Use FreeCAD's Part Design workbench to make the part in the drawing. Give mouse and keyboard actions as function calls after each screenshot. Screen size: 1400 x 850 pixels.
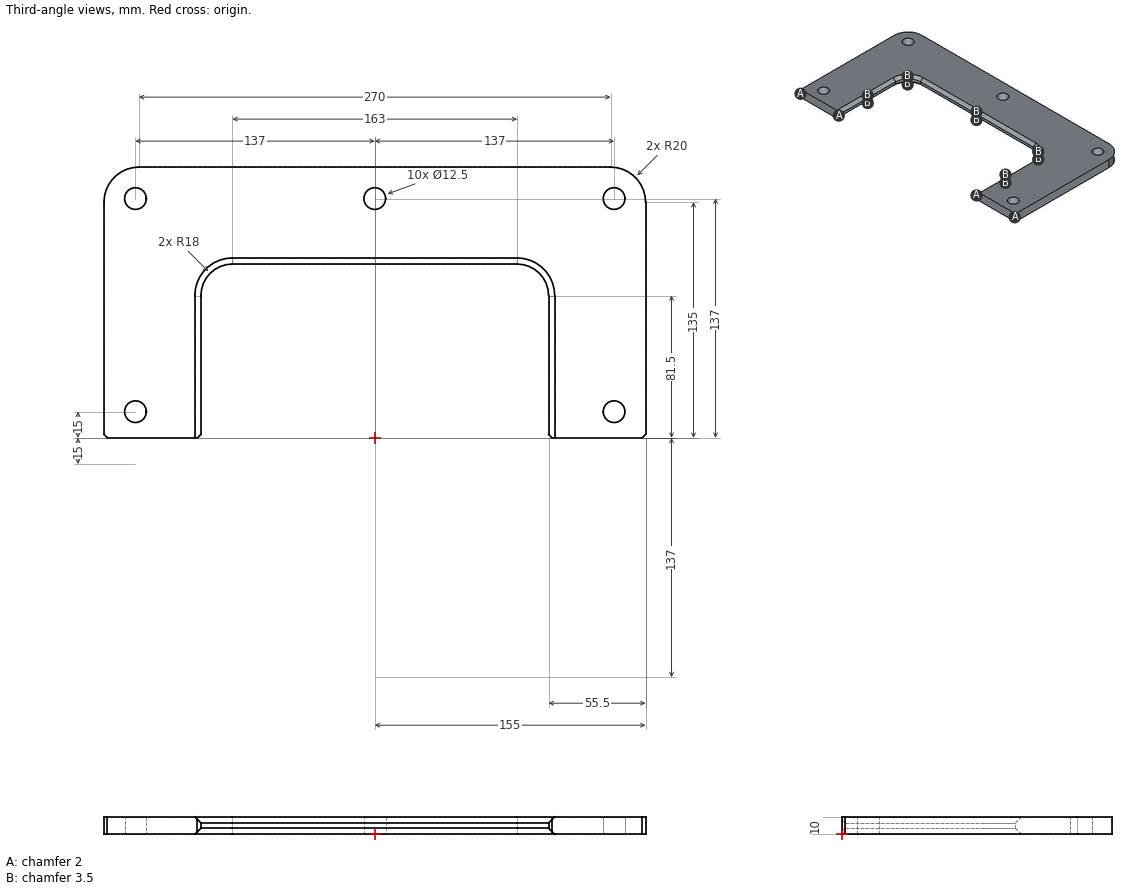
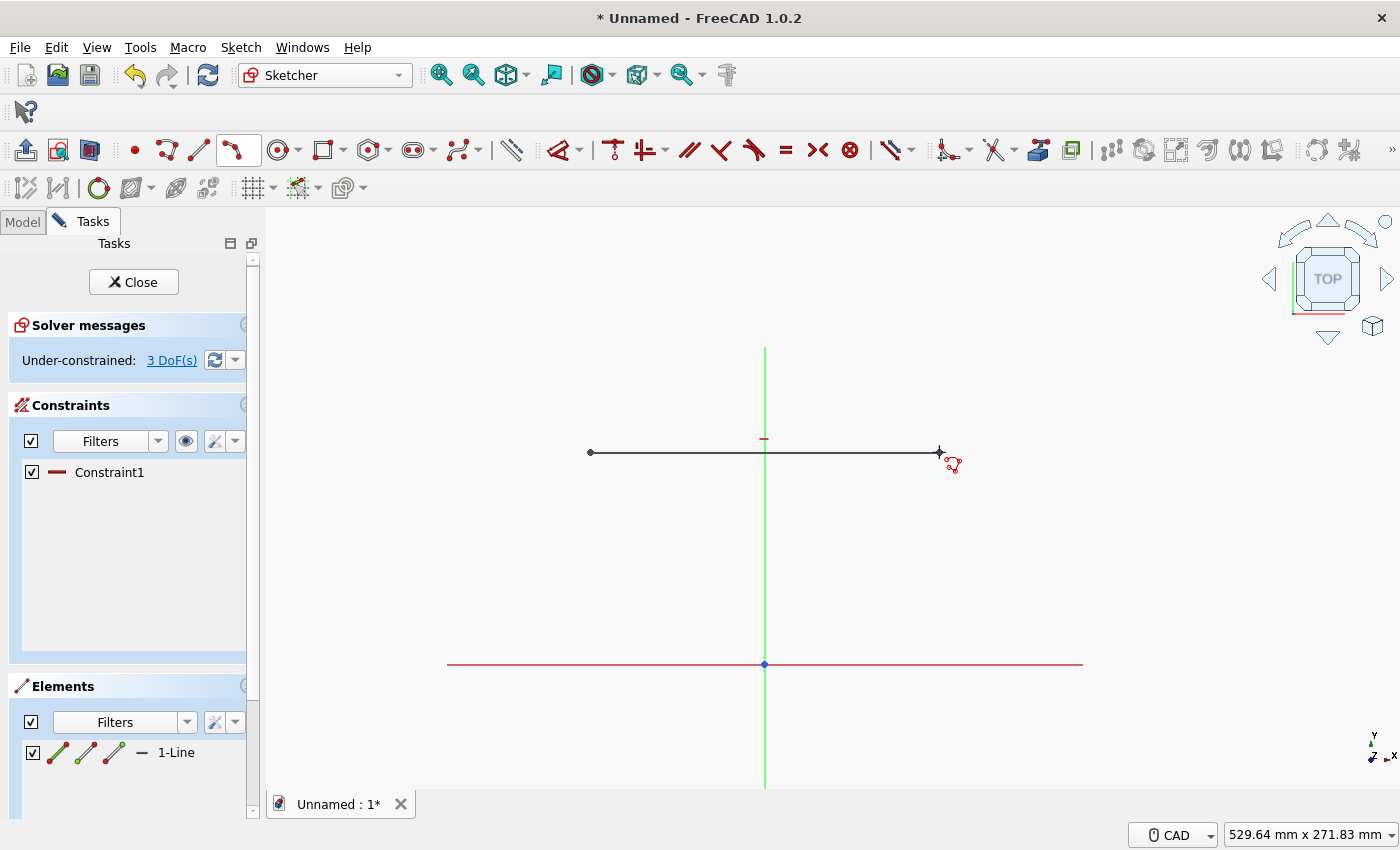
click(978, 490)
click(978, 665)
click(1097, 656)
click(1097, 376)
right_click(1097, 376)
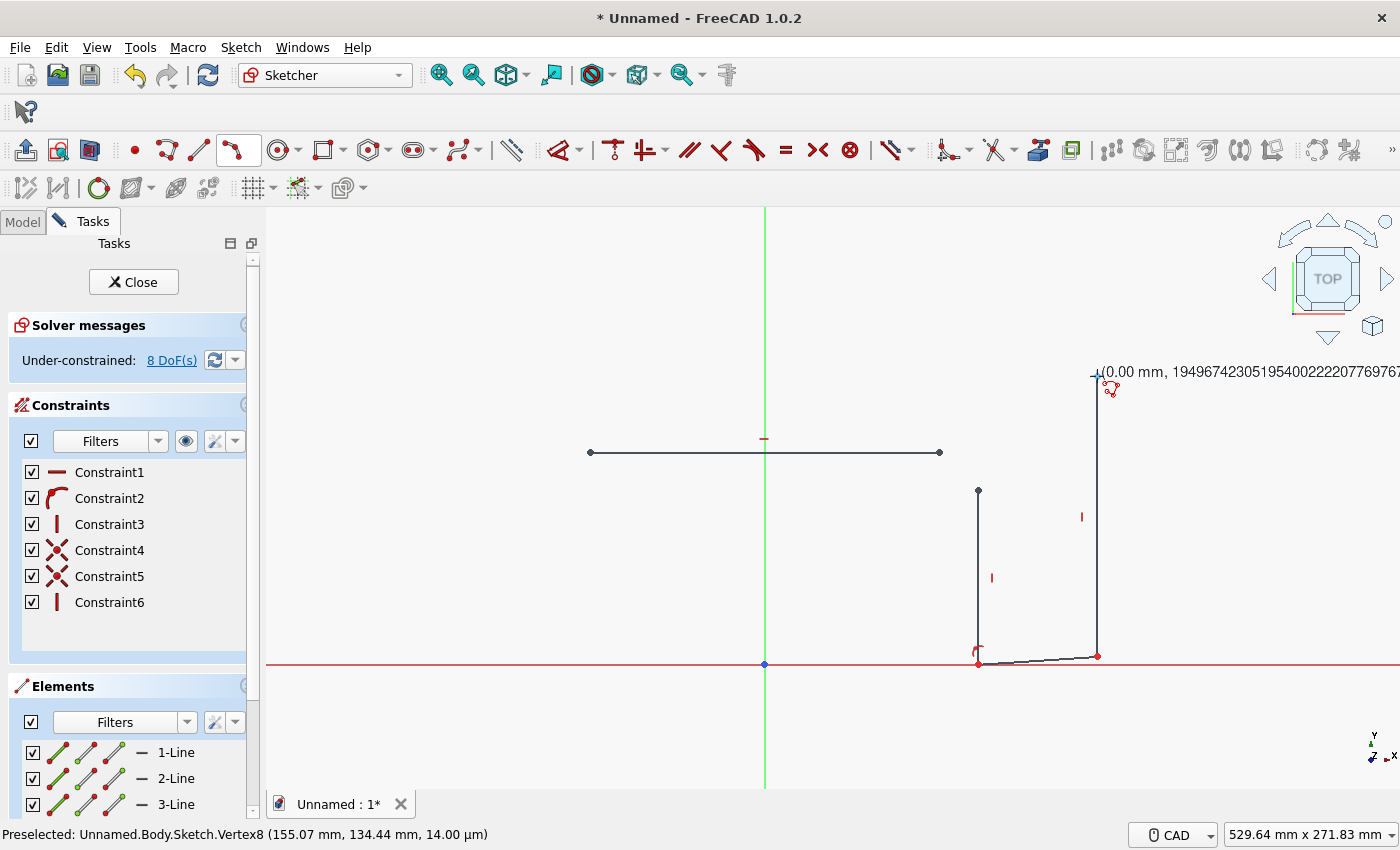
click(200, 150)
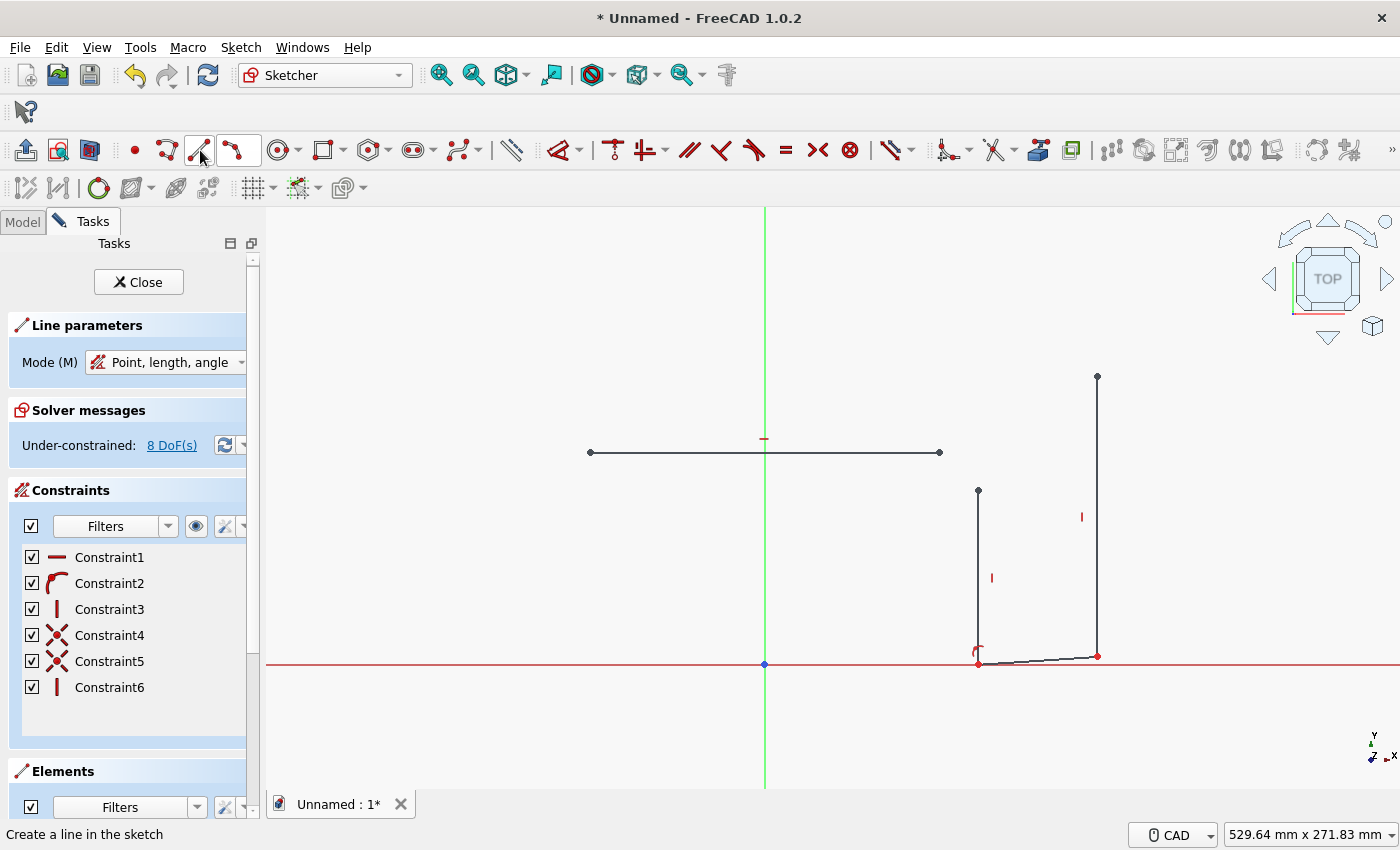
click(1054, 333)
click(476, 333)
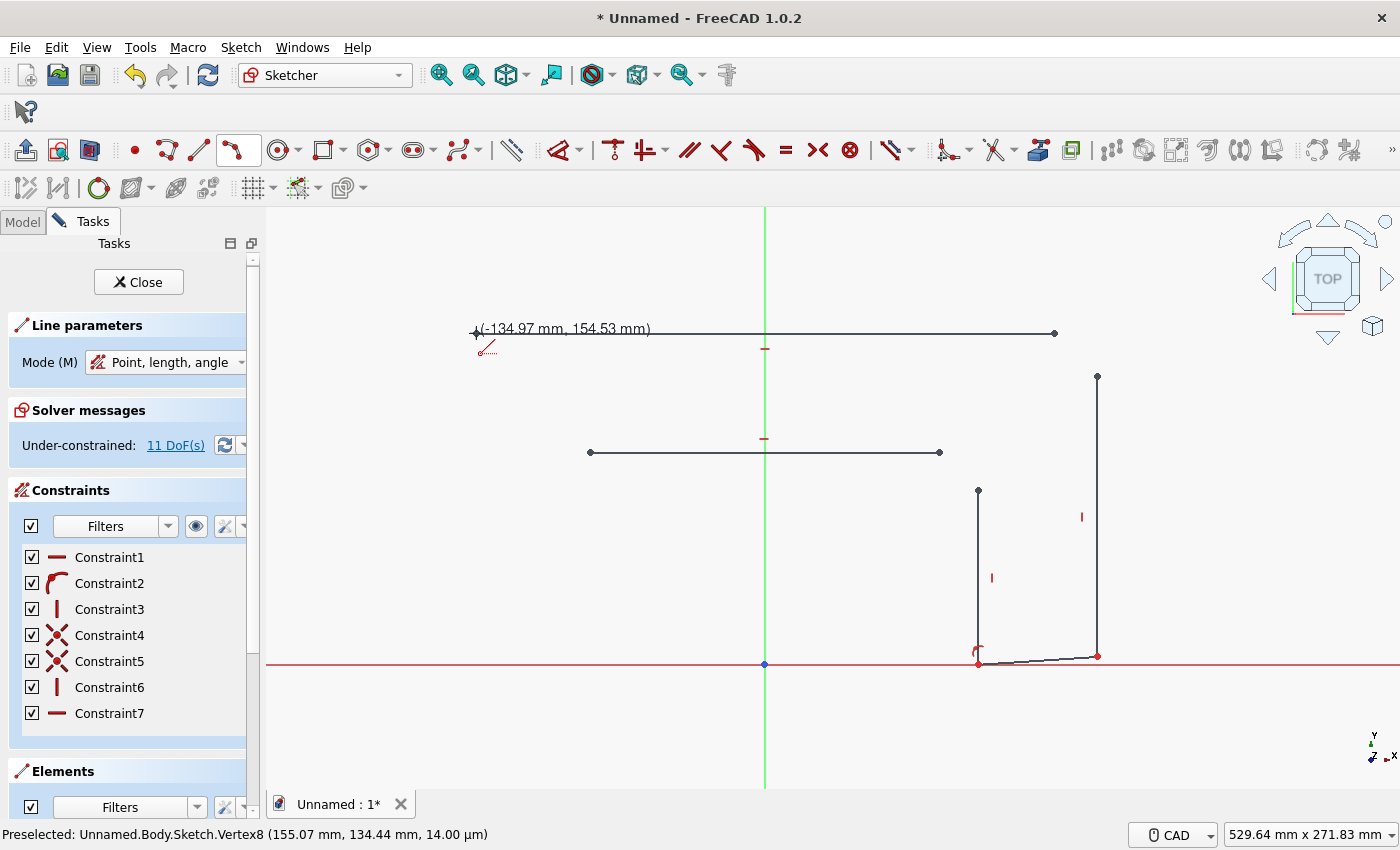
key(g)
key(m)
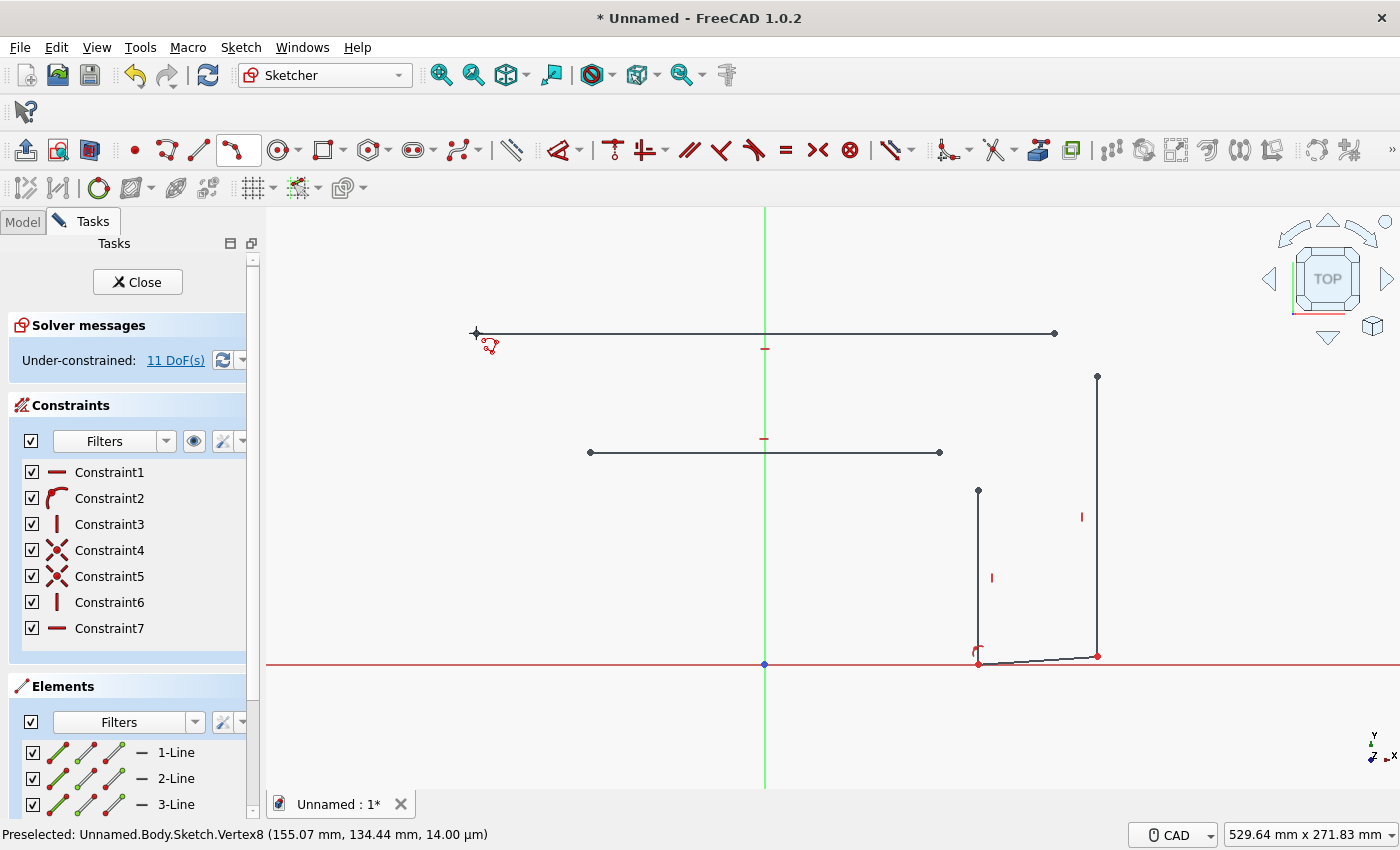
click(433, 376)
click(433, 665)
click(552, 656)
click(552, 490)
right_click(552, 490)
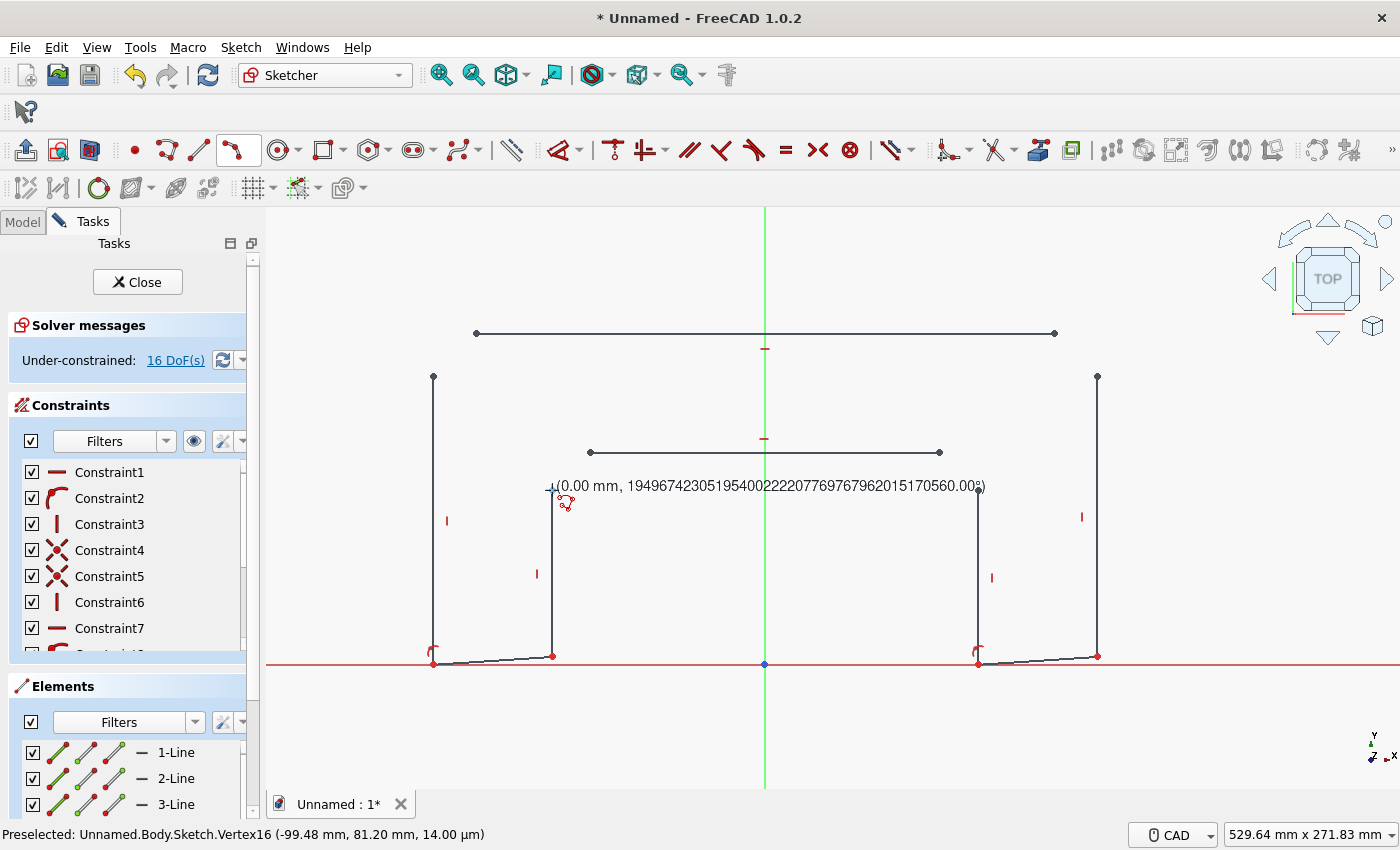
key(g)
key(3)
key(a)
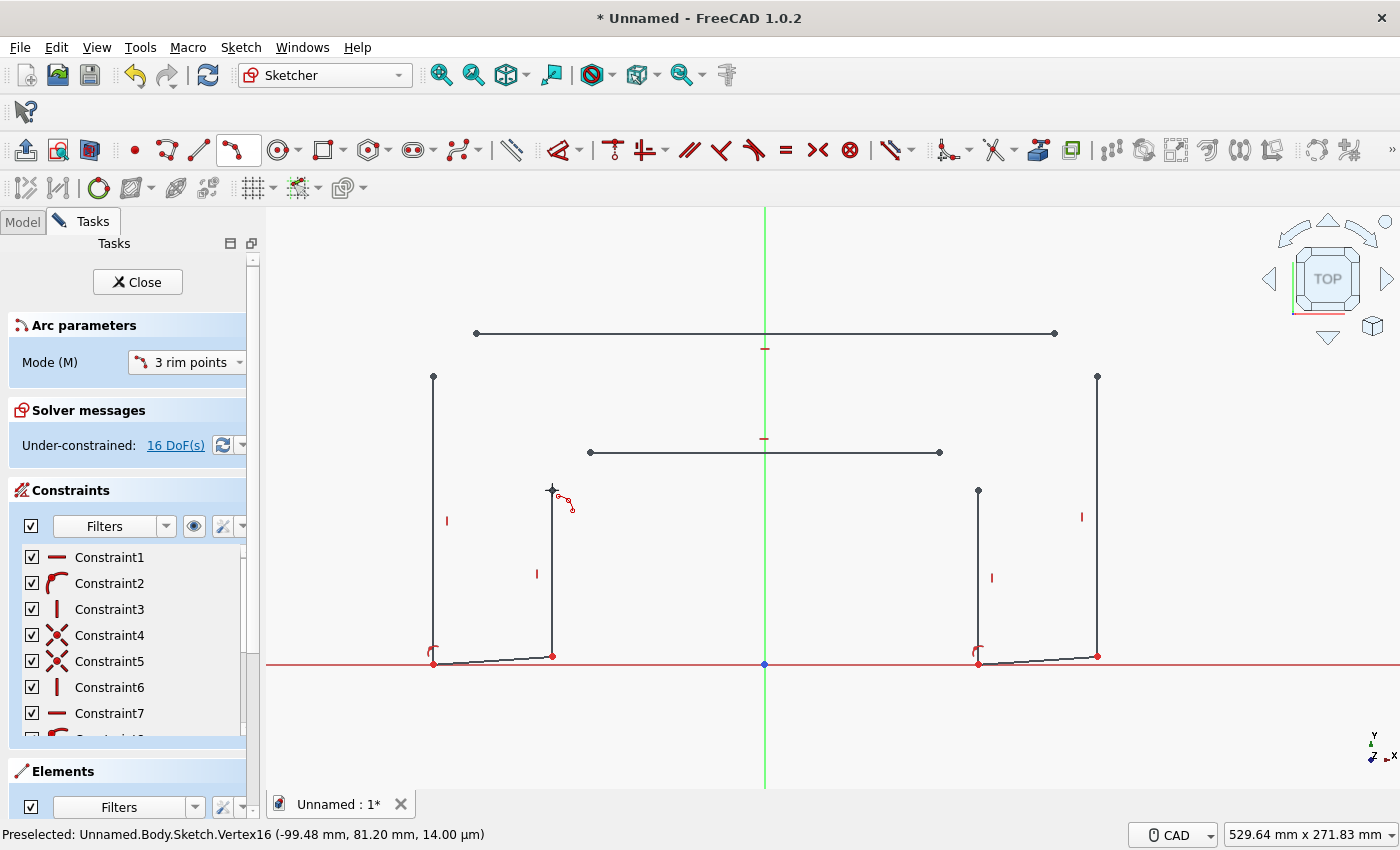
click(939, 453)
click(978, 491)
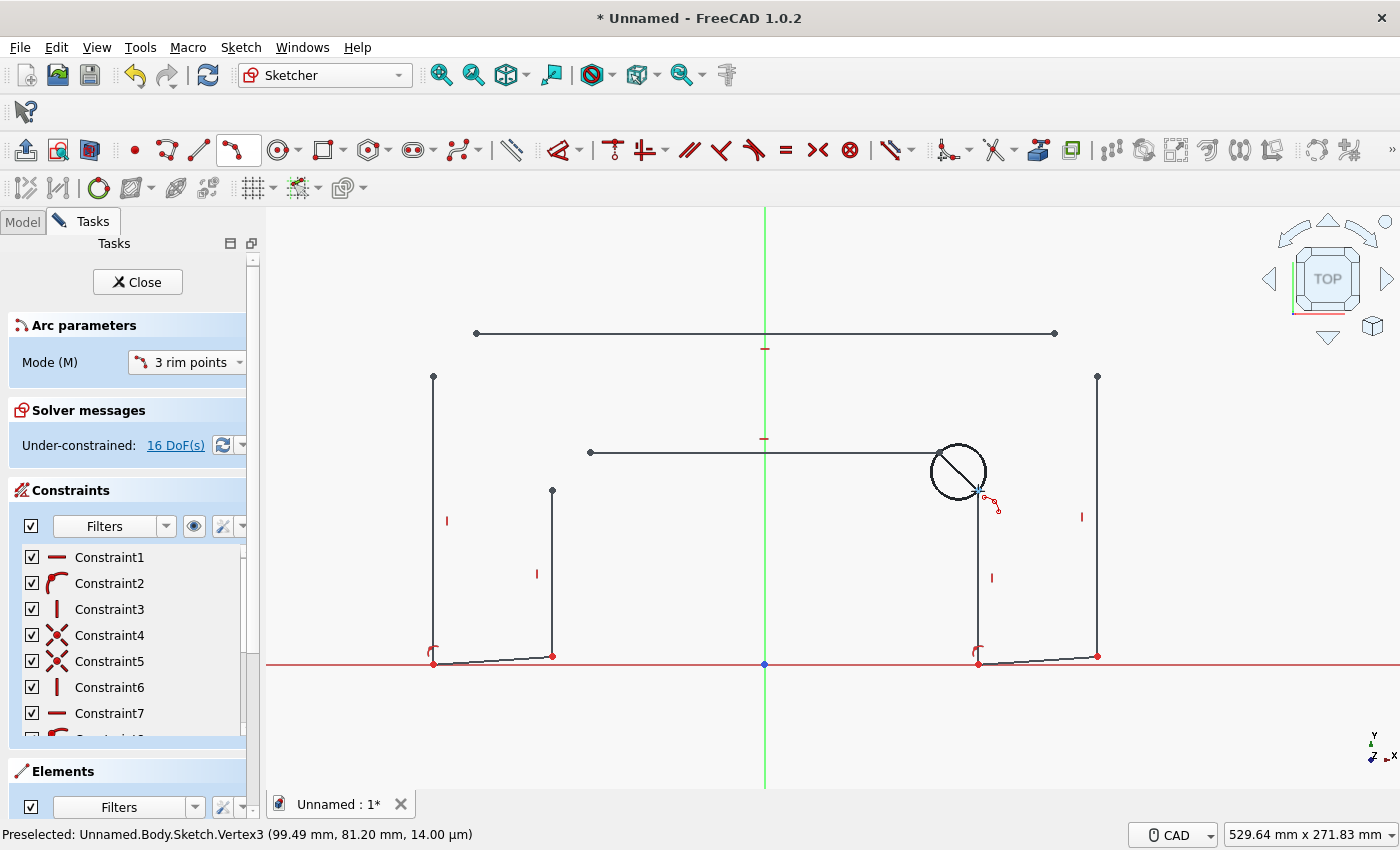
scroll(967, 463, up, 2)